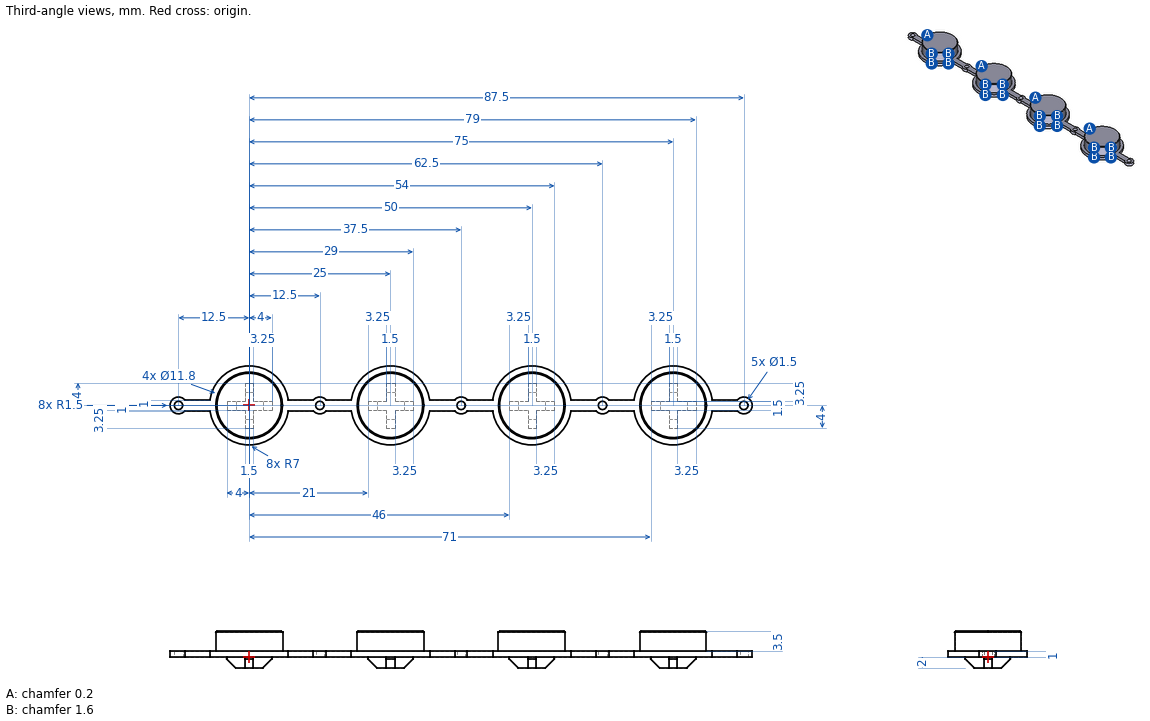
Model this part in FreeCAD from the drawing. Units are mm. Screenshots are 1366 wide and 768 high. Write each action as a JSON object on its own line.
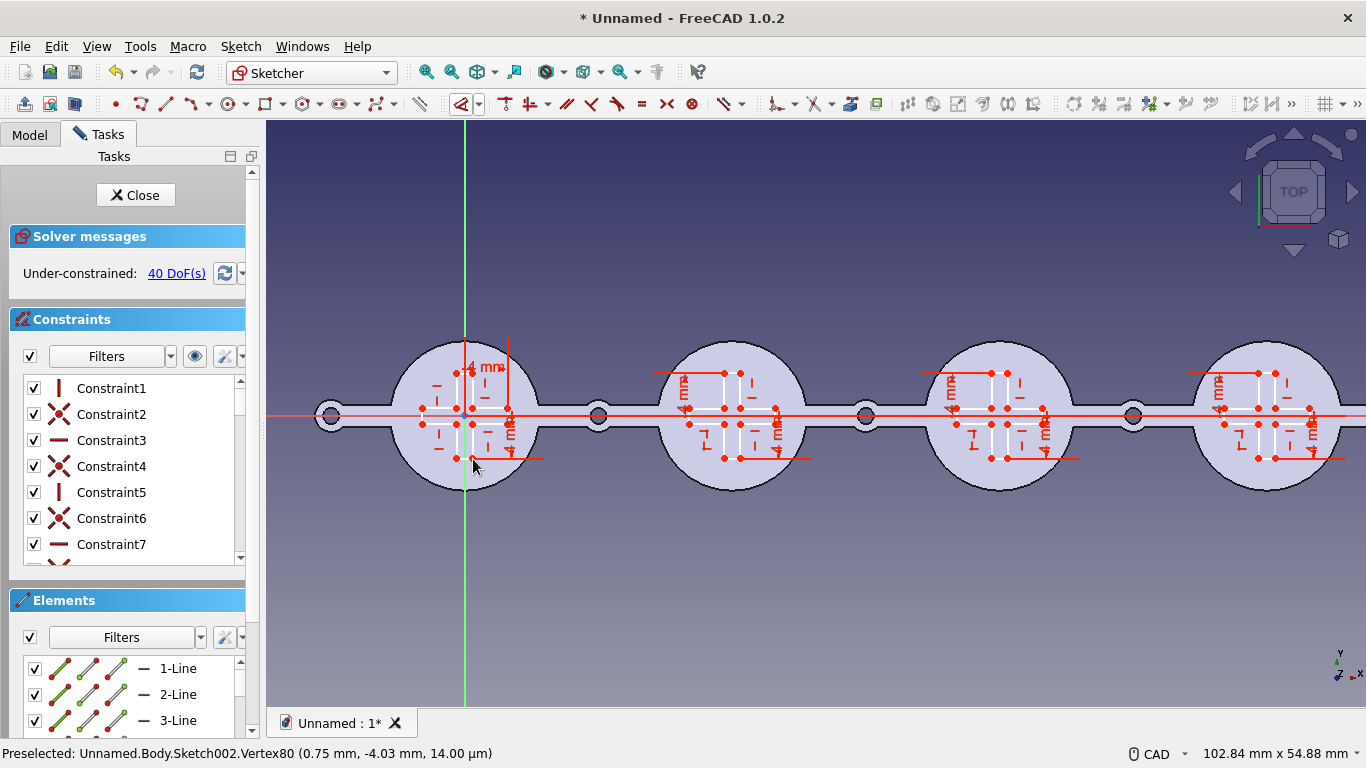
{"action": "left_click", "coordinate": [422, 424]}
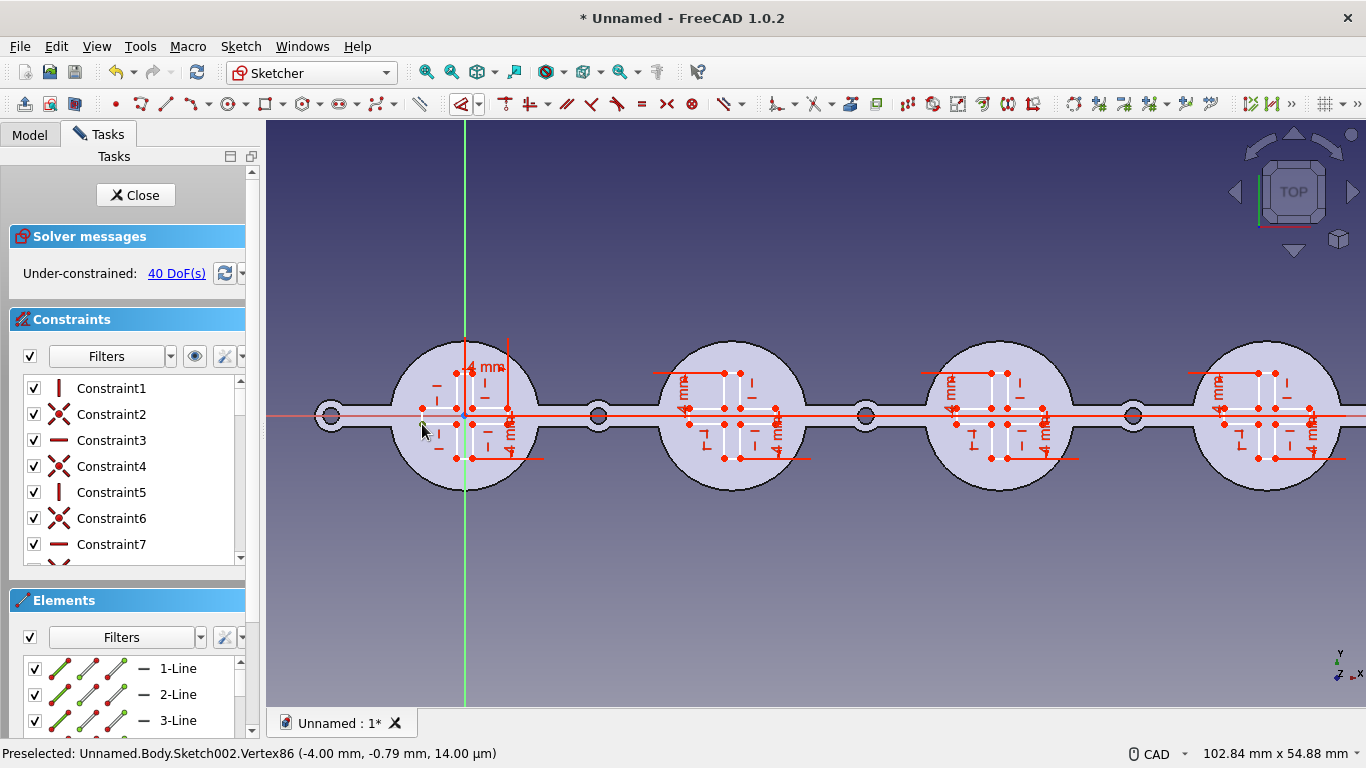
{"action": "key", "text": "l"}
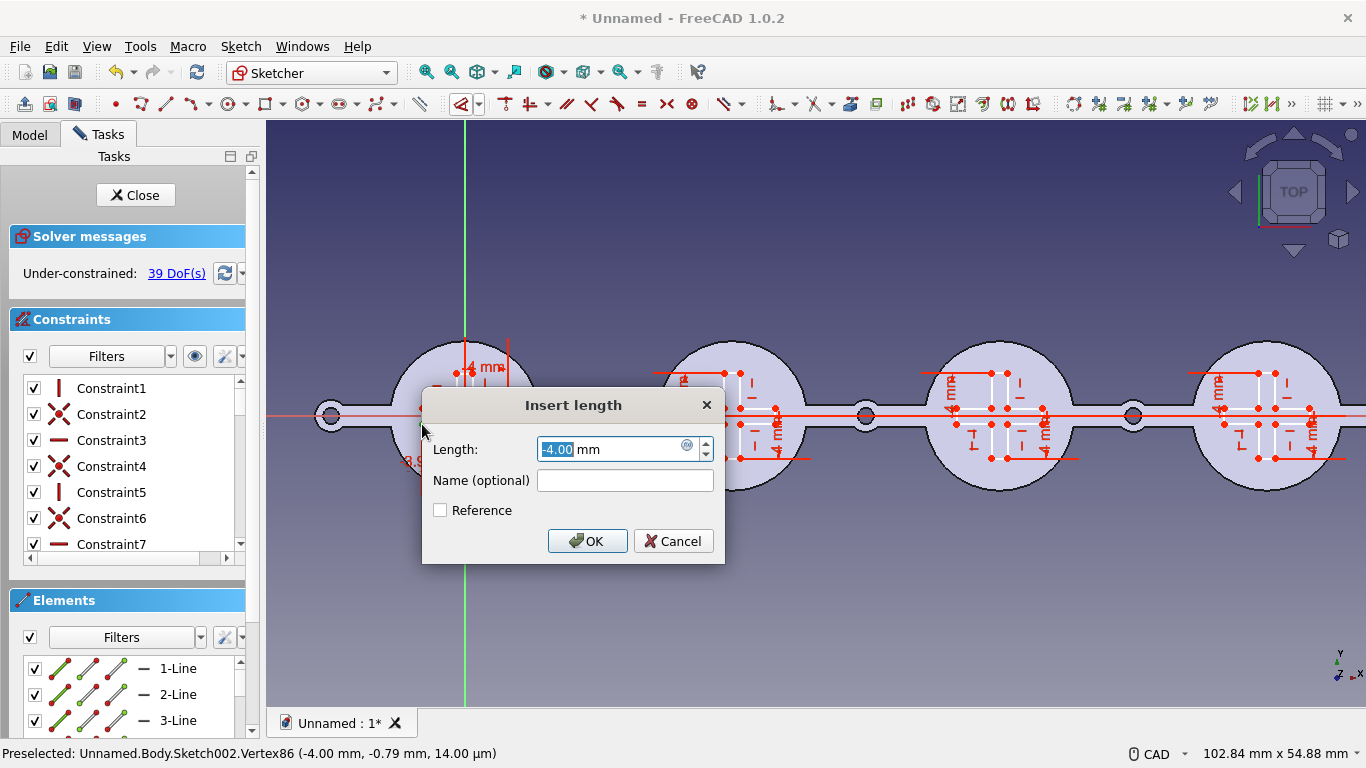
{"action": "type", "text": "-4"}
{"action": "key", "text": "Return"}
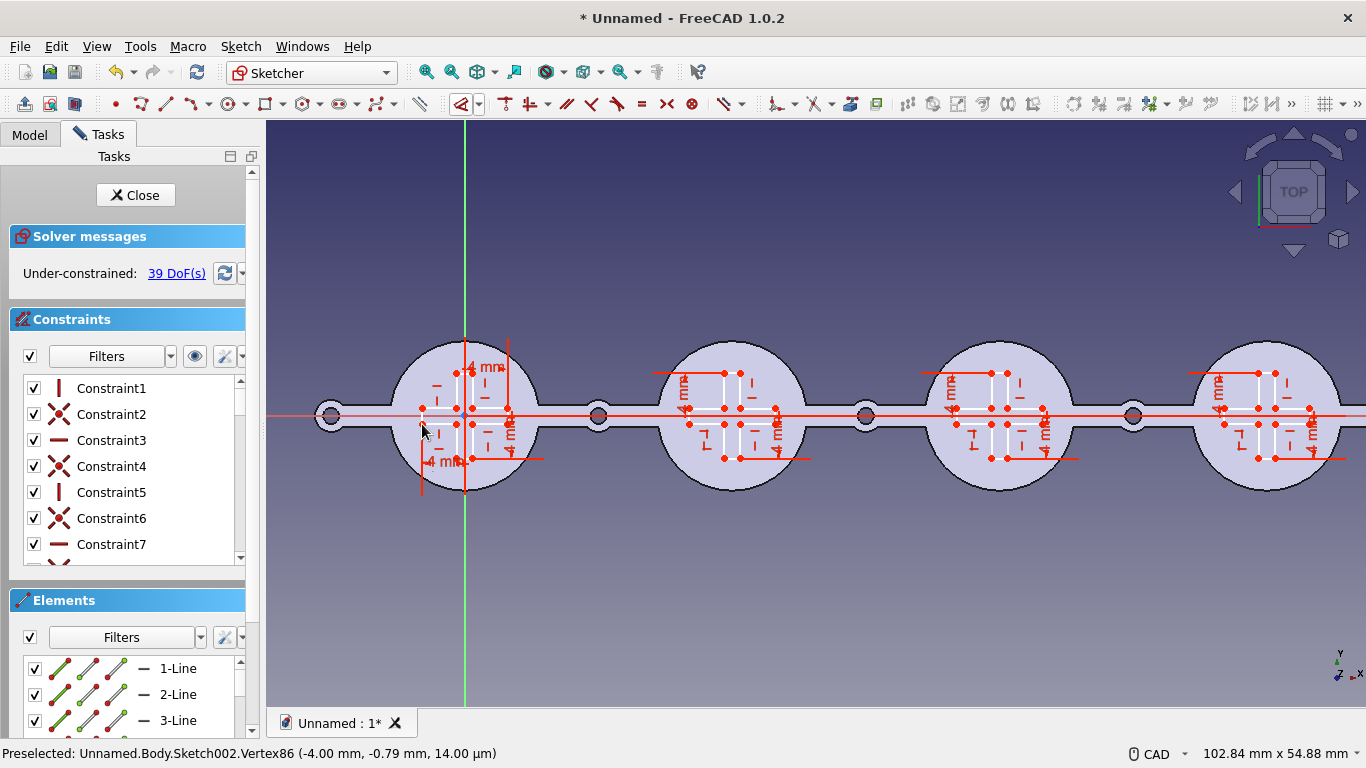
{"action": "left_click", "coordinate": [457, 374]}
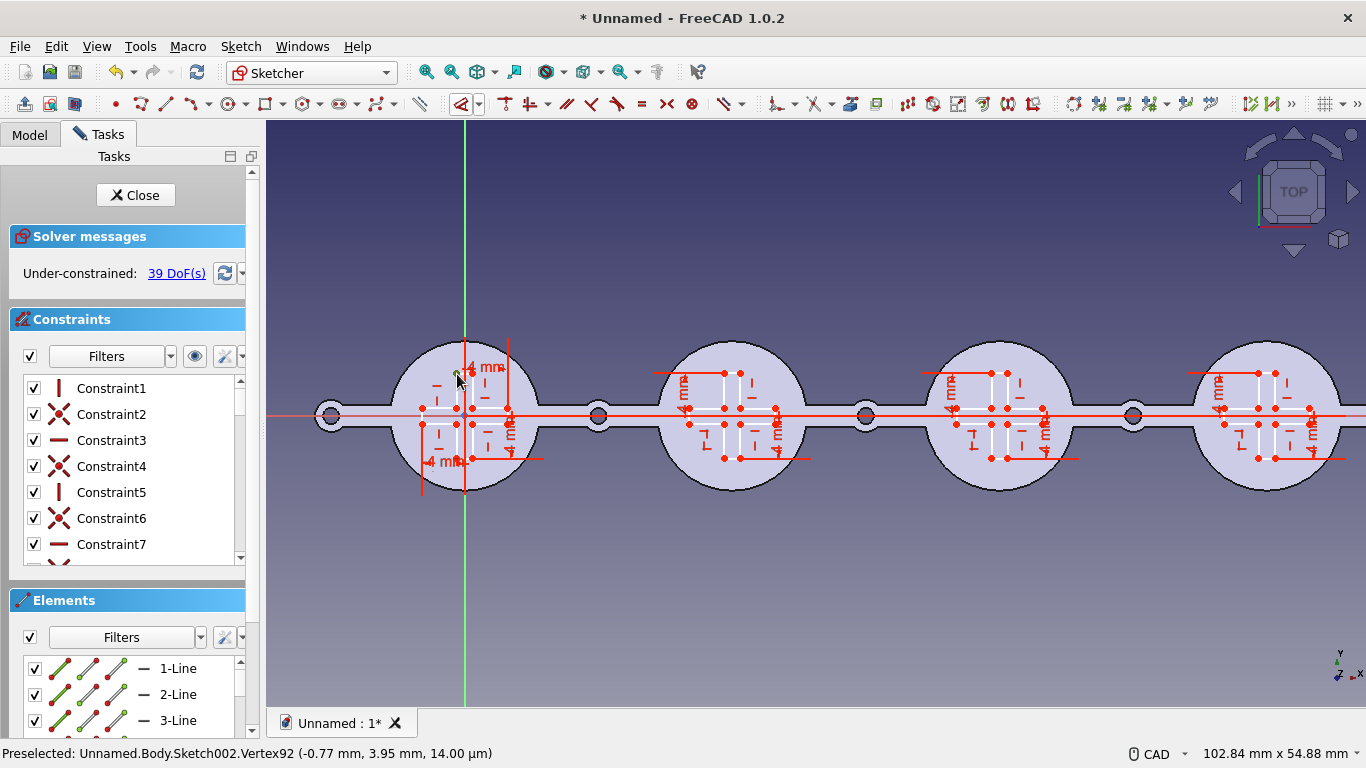
{"action": "left_click", "coordinate": [478, 104]}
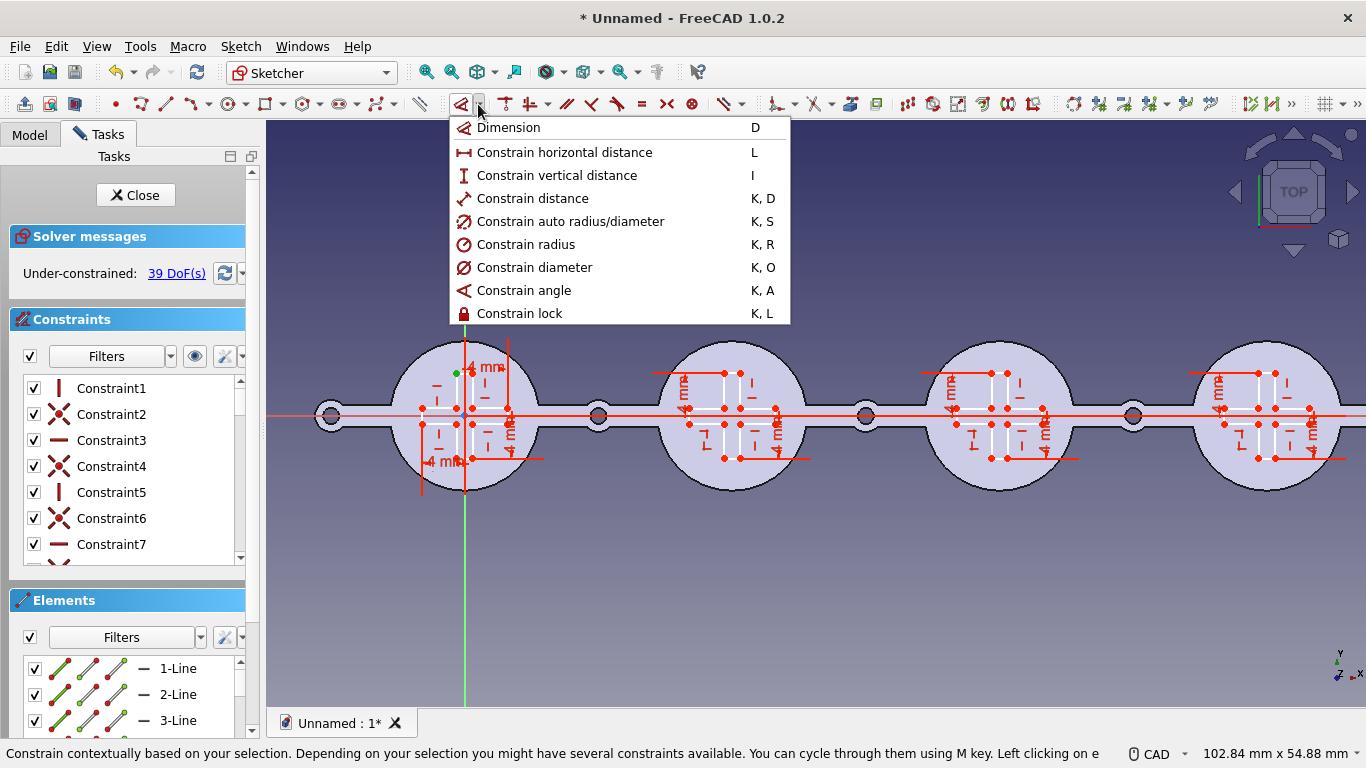
{"action": "left_click", "coordinate": [620, 176]}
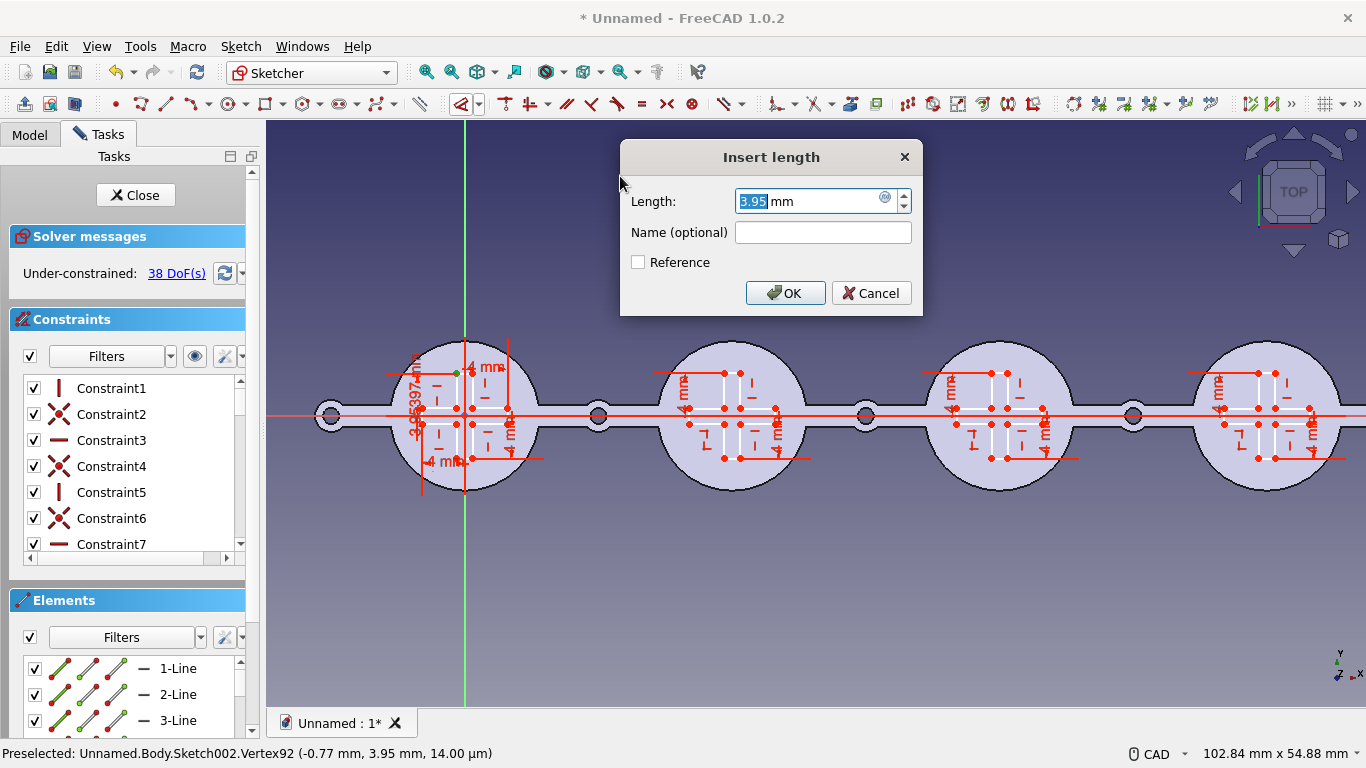
{"action": "type", "text": "4"}
{"action": "key", "text": "Return"}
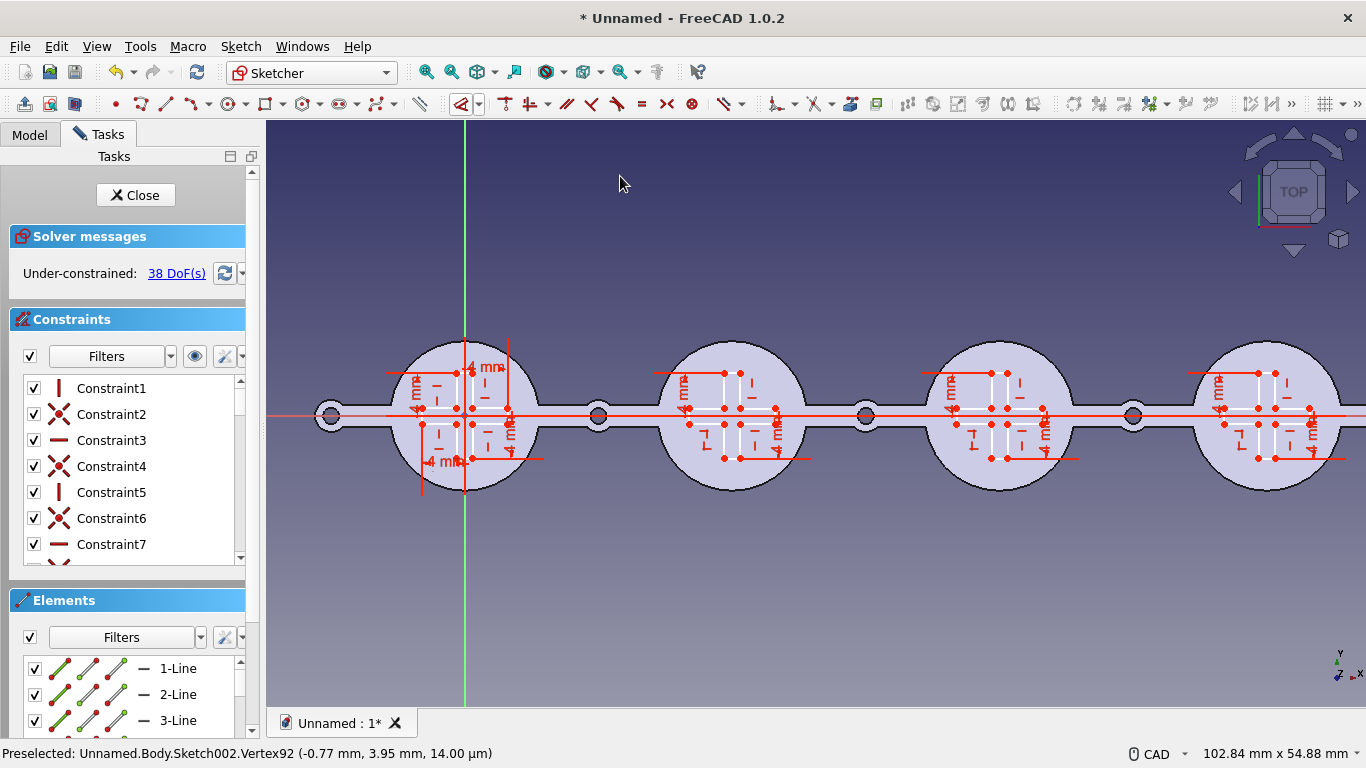
{"action": "scroll", "coordinate": [507, 408], "scroll_direction": "down", "scroll_amount": 2}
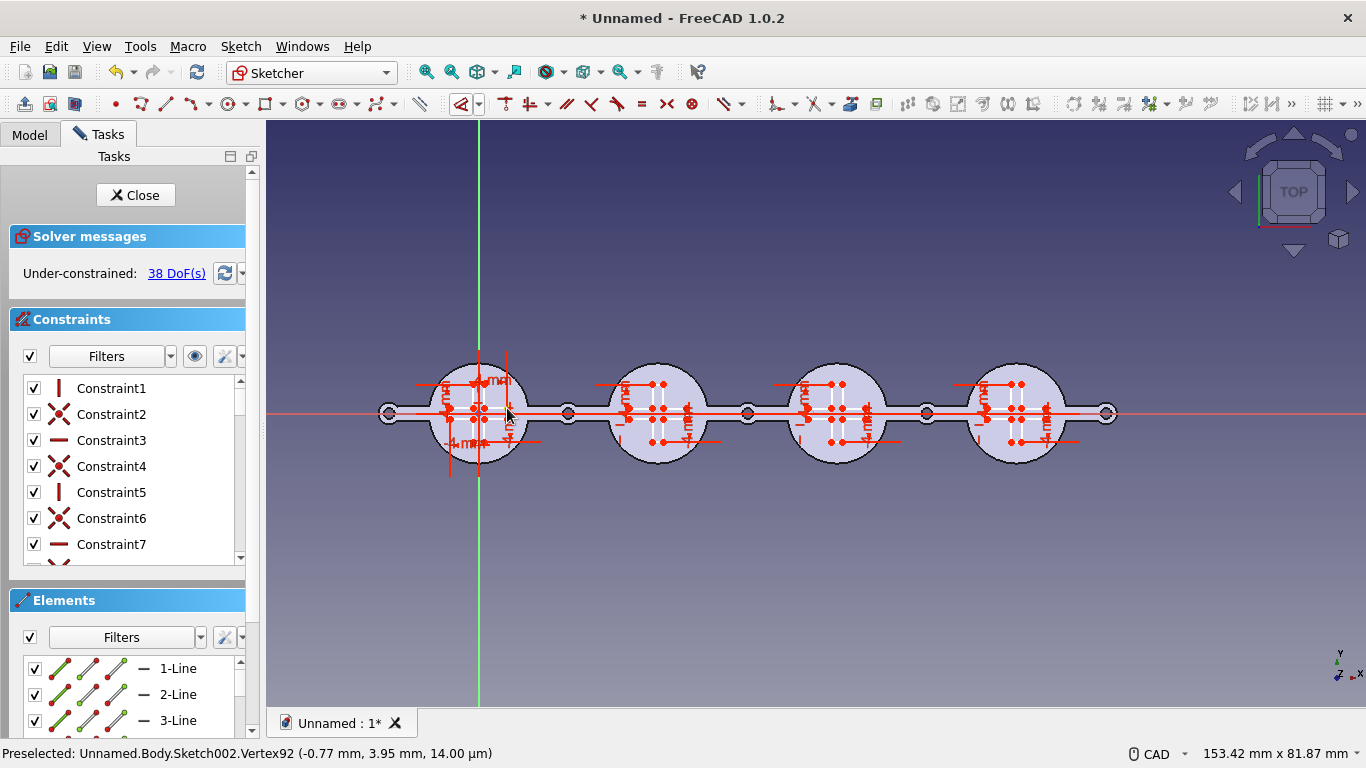
{"action": "scroll", "coordinate": [988, 414], "scroll_direction": "up", "scroll_amount": 7}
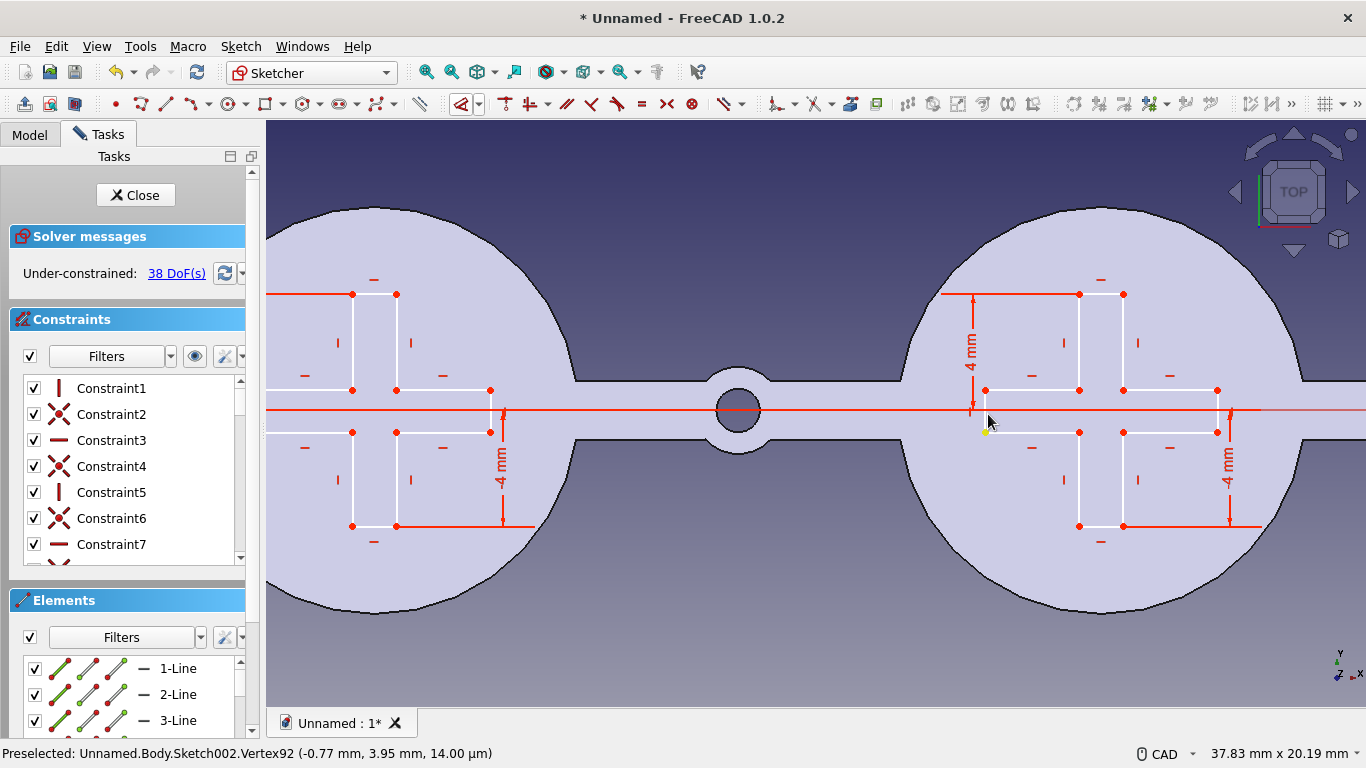
{"action": "left_click", "coordinate": [985, 412]}